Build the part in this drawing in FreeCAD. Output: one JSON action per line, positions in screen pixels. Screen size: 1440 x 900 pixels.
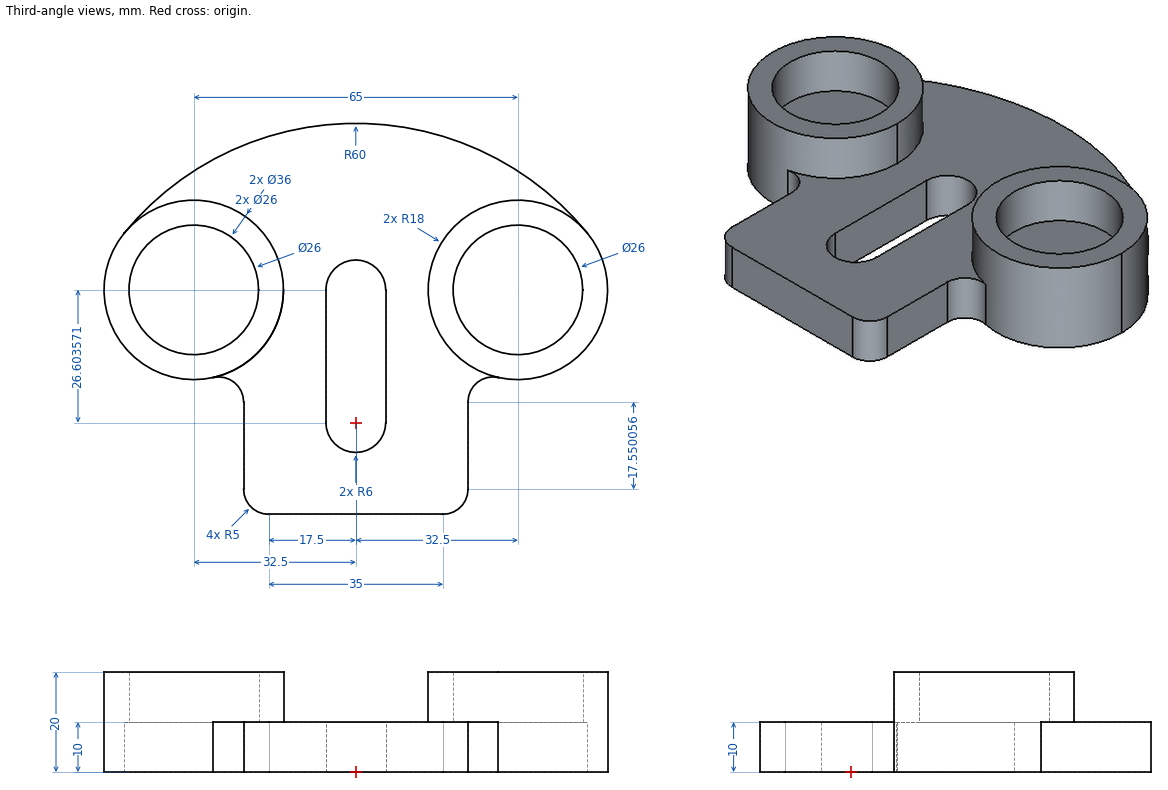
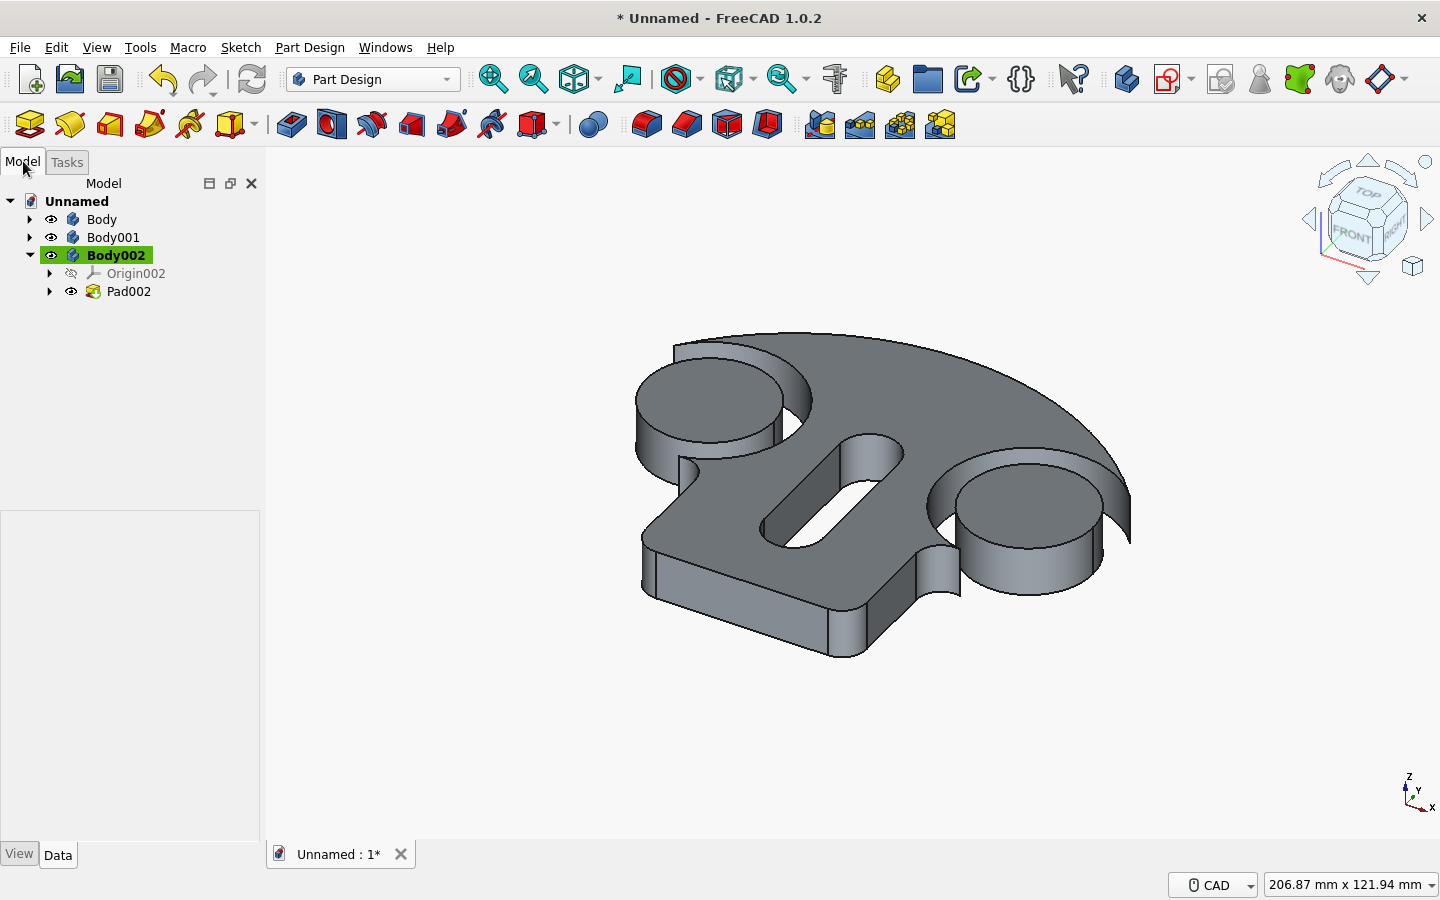
{"action": "double_click", "coordinate": [96, 219]}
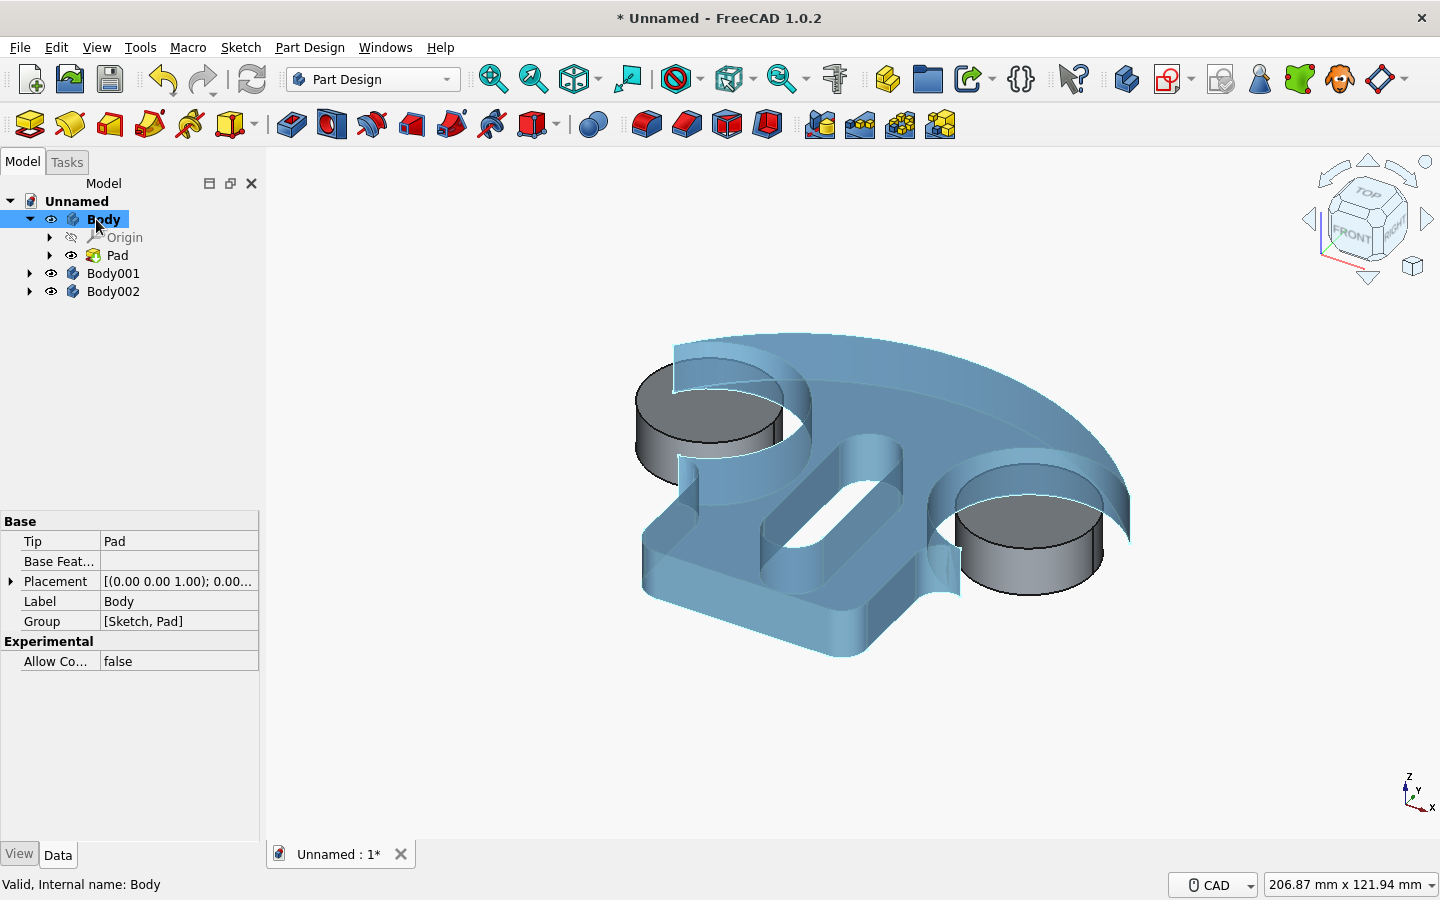
{"action": "left_click", "coordinate": [96, 219]}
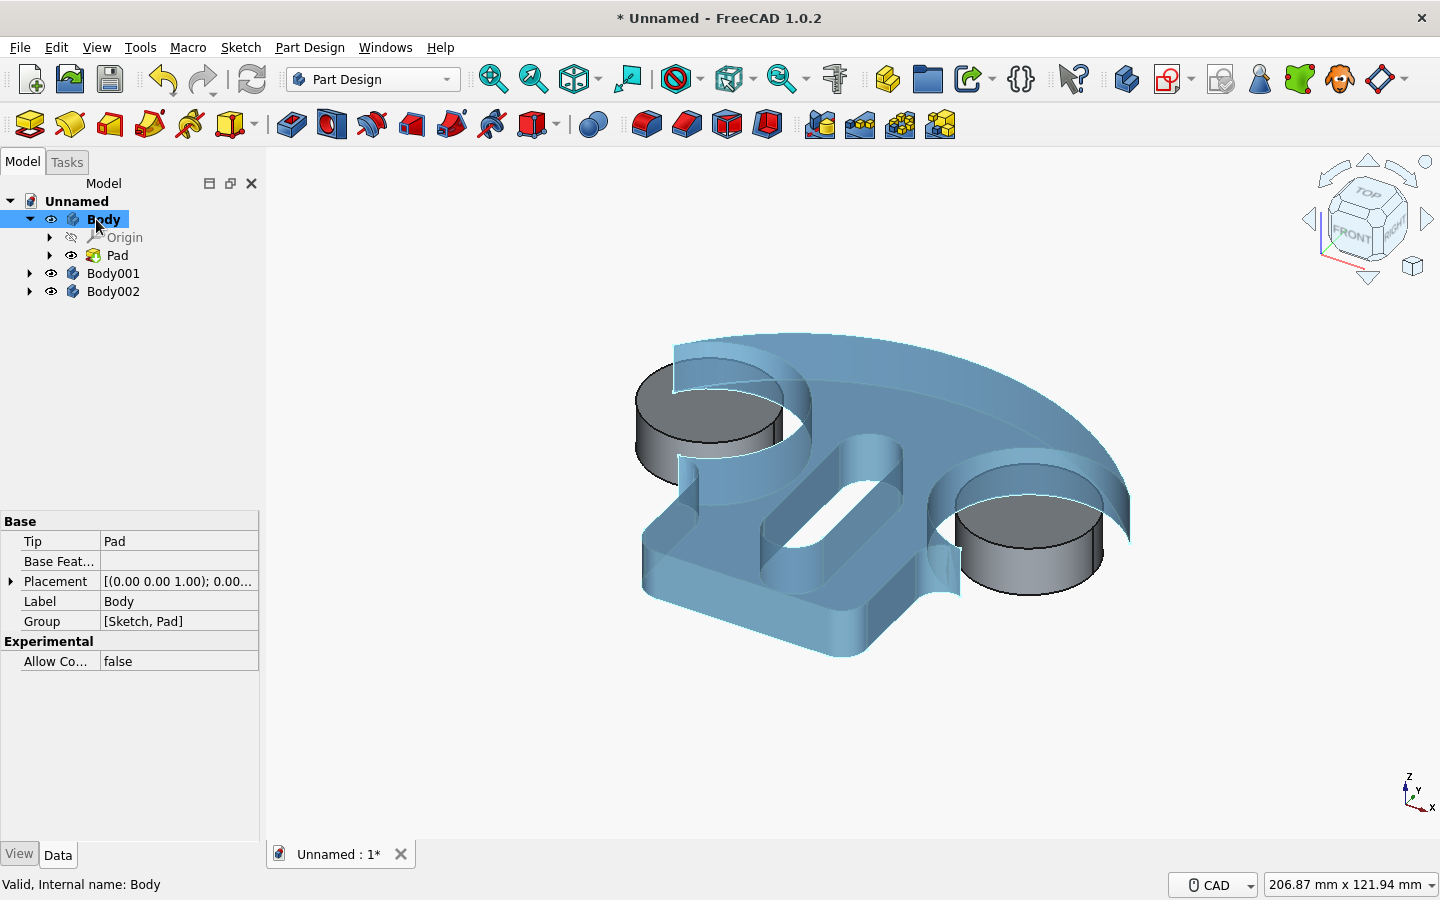
{"action": "left_click", "coordinate": [146, 661]}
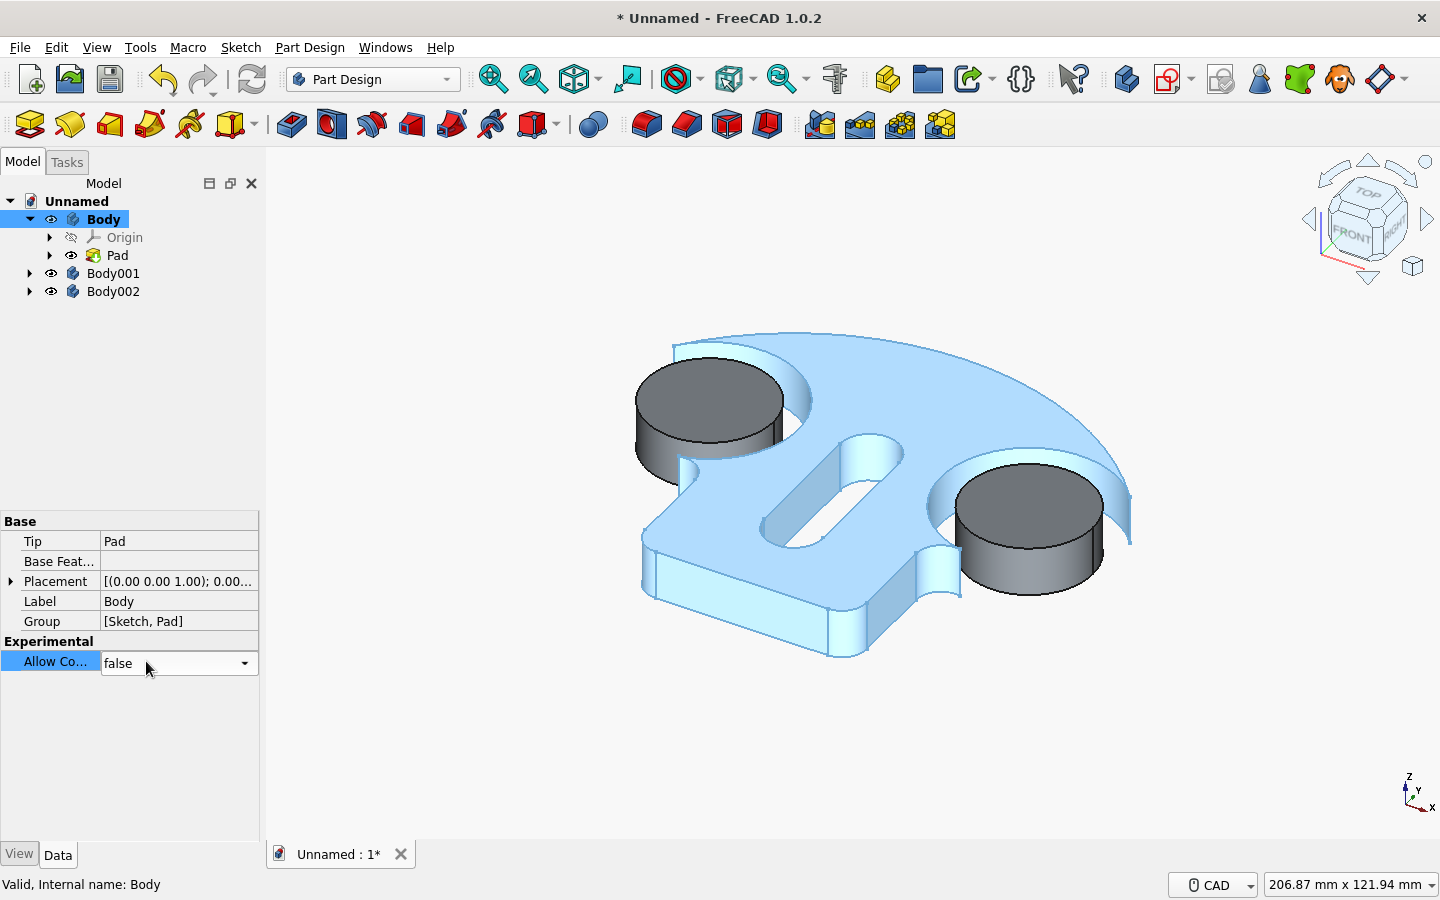
{"action": "left_click", "coordinate": [146, 661]}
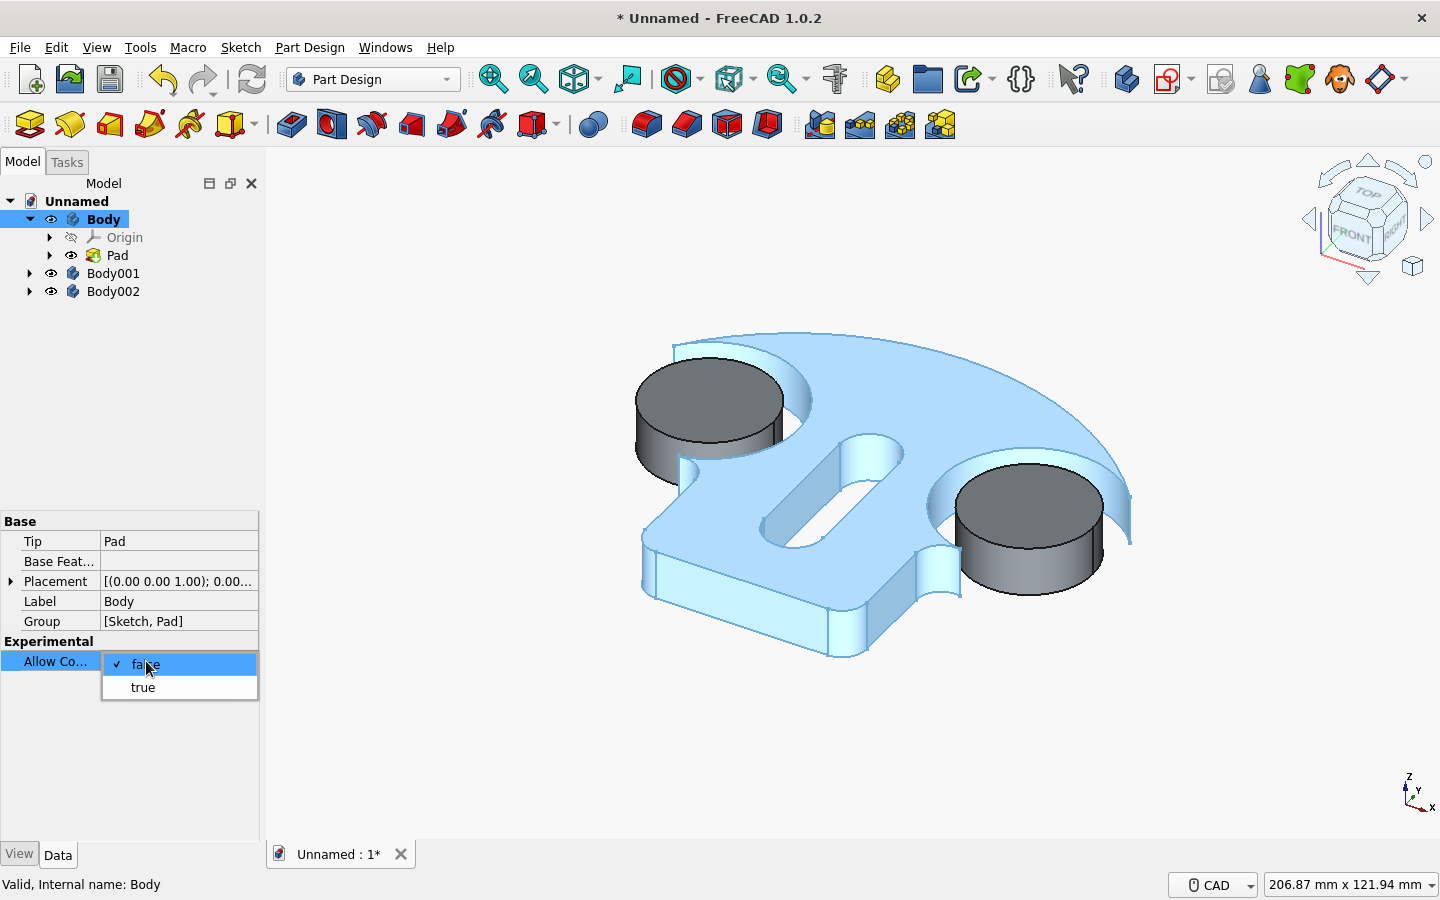
{"action": "left_click", "coordinate": [179, 688]}
{"action": "key", "text": "Return"}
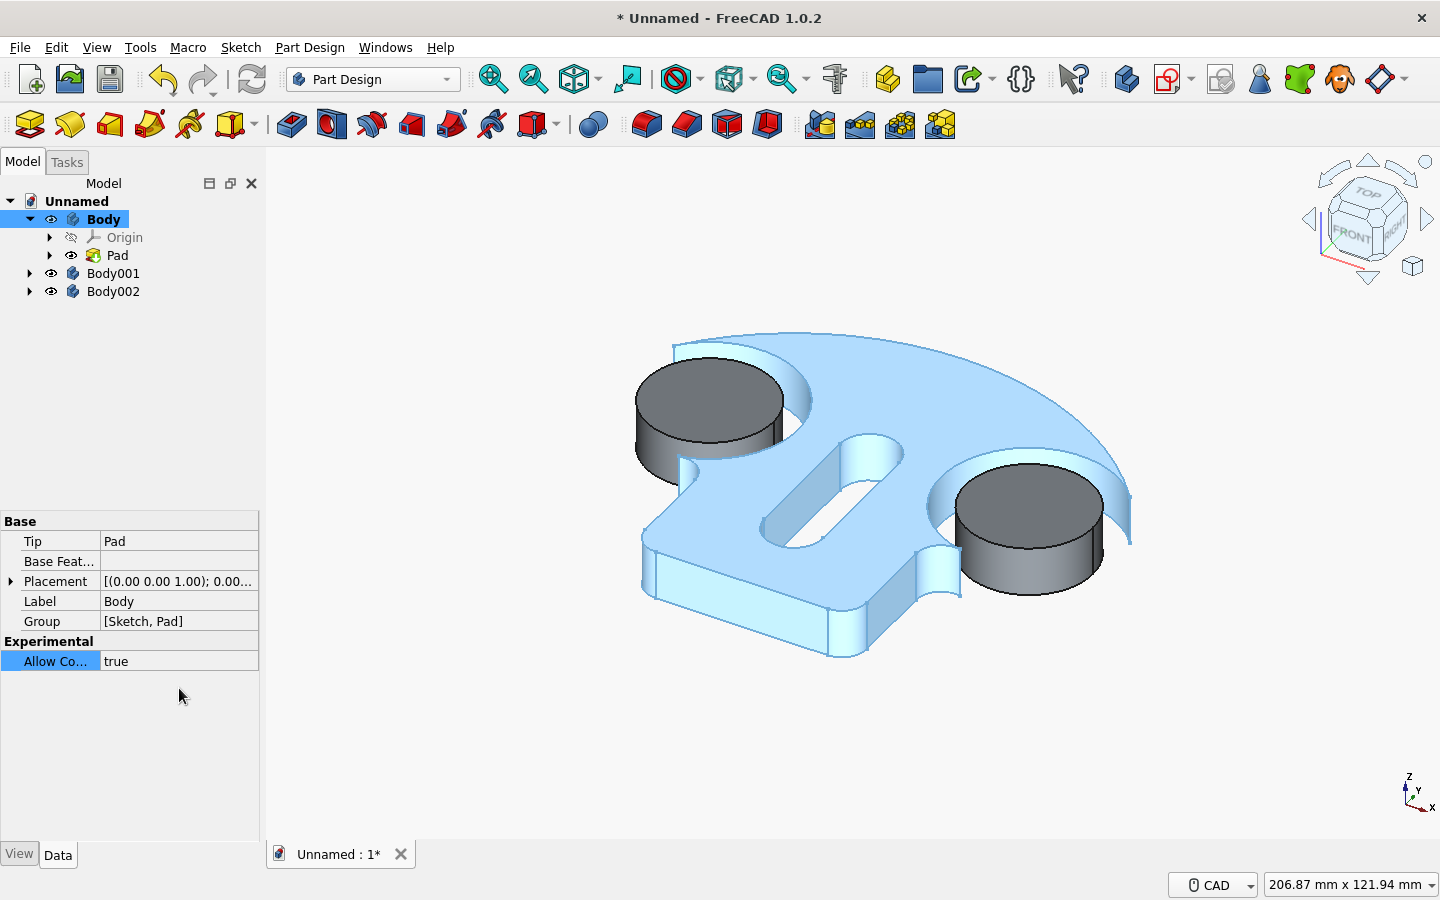
{"action": "left_click", "coordinate": [96, 273]}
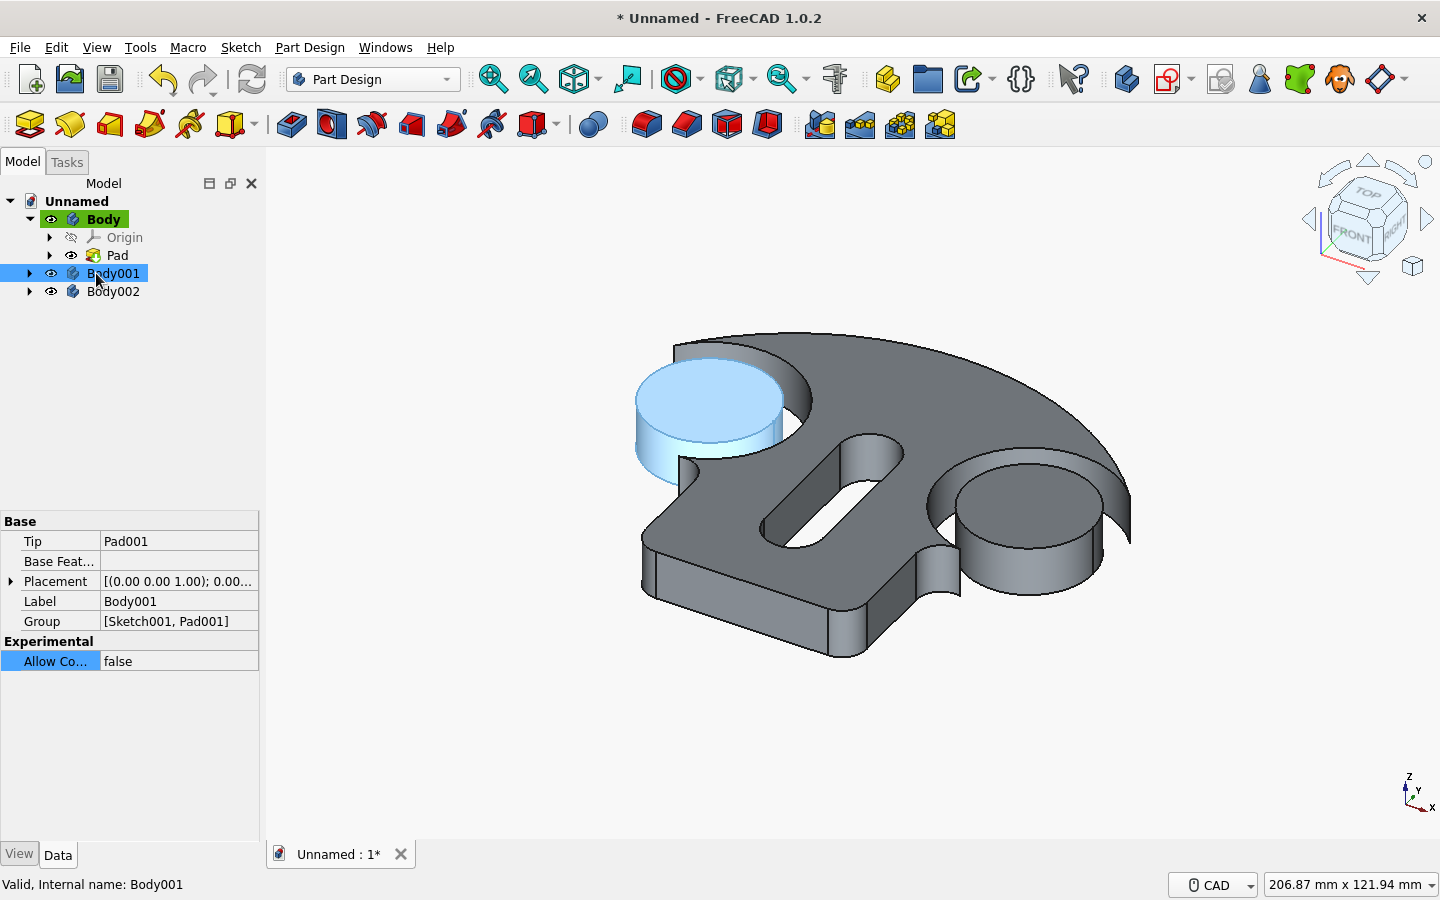
{"action": "left_click", "coordinate": [594, 124]}